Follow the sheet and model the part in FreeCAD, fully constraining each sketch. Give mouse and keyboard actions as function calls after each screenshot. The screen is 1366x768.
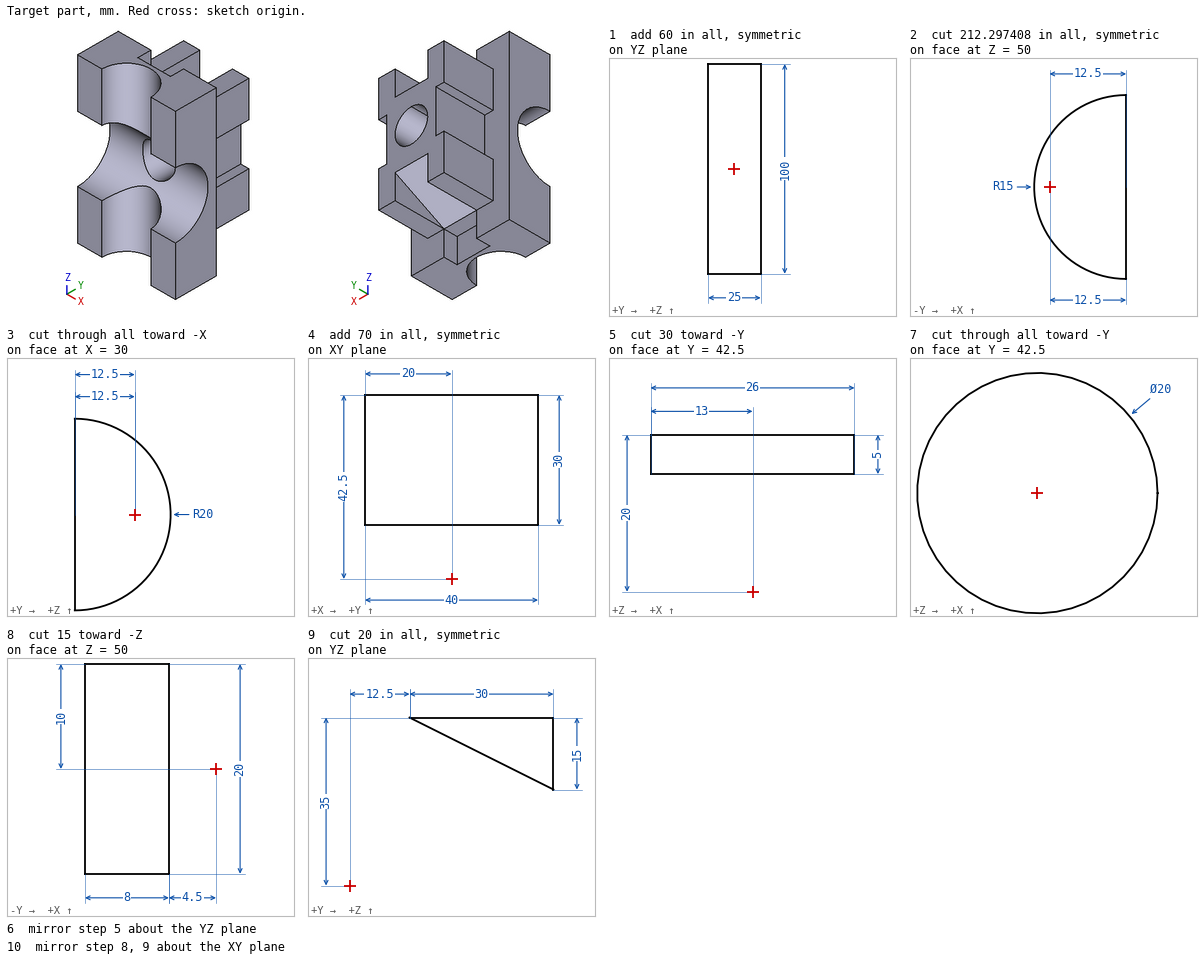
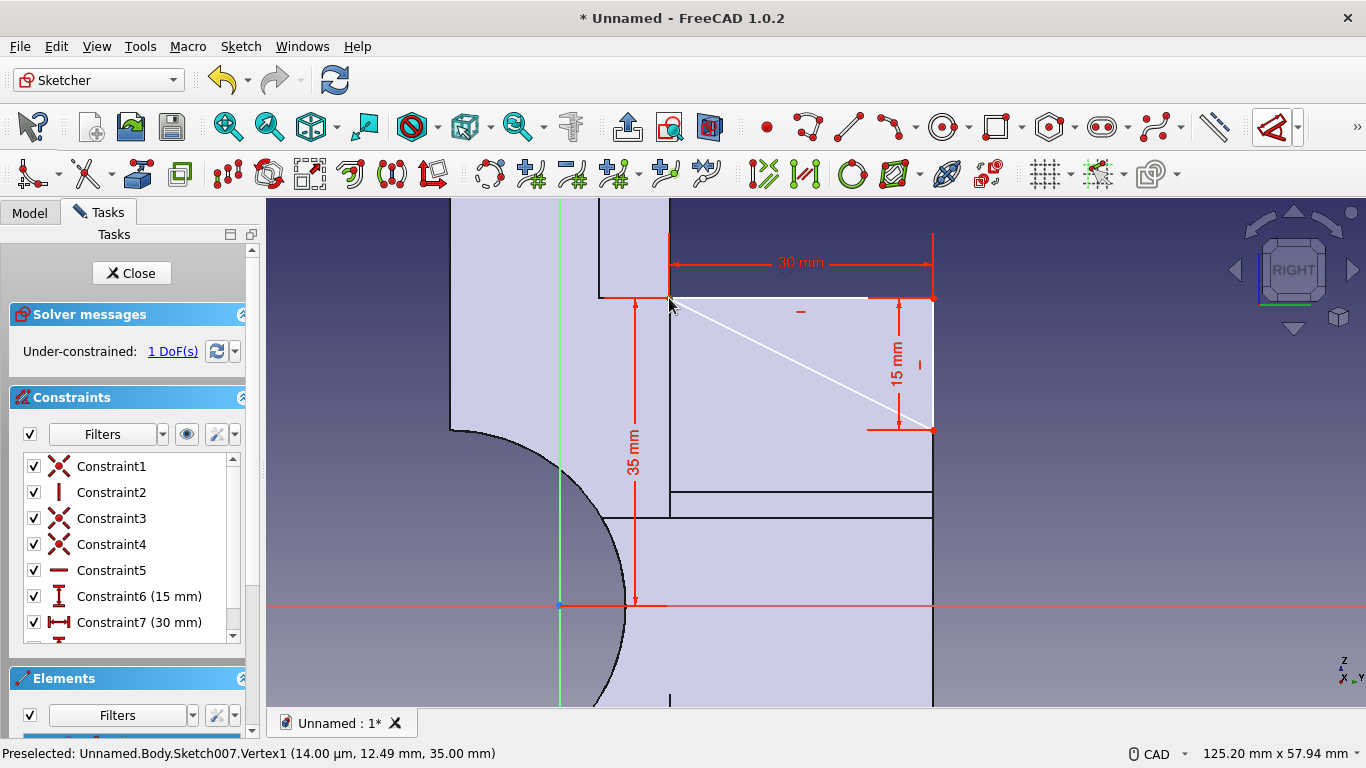
key(l)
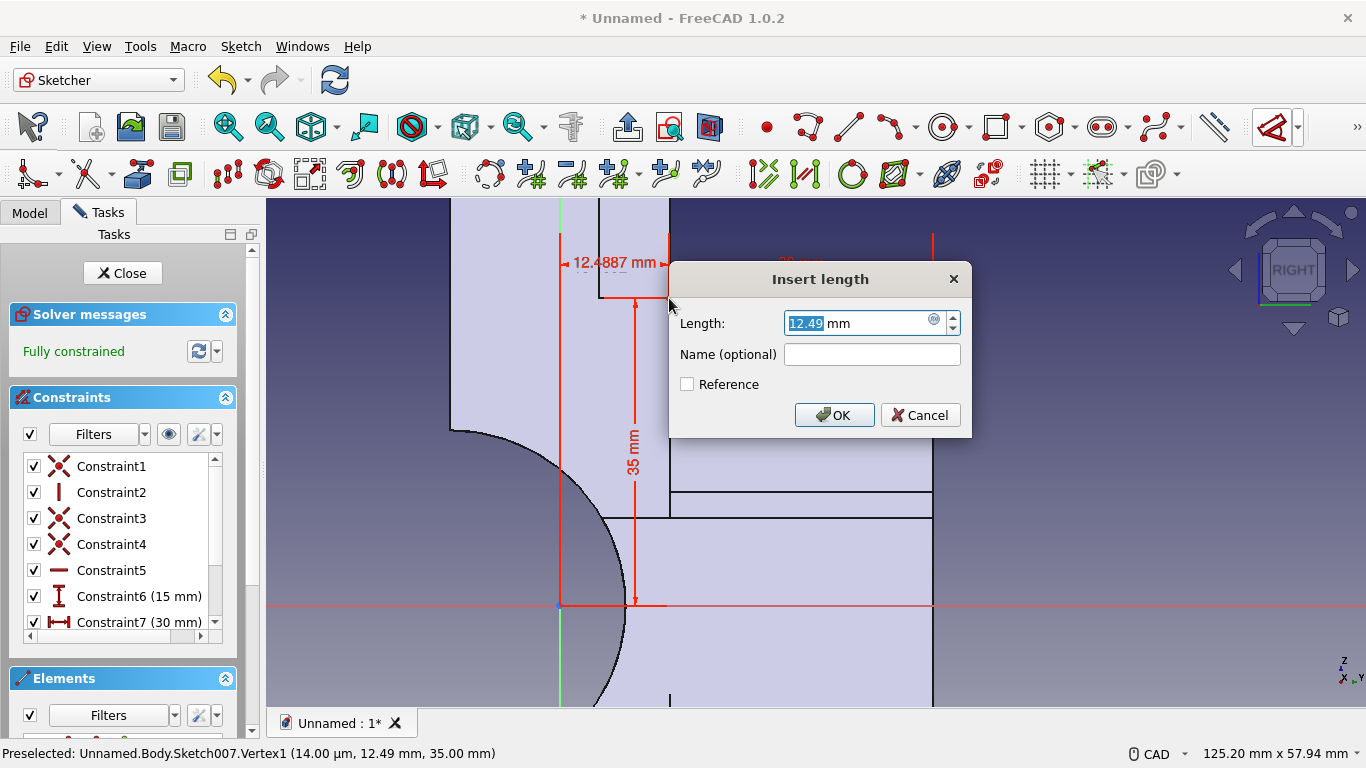
text(12.5)
key(Return)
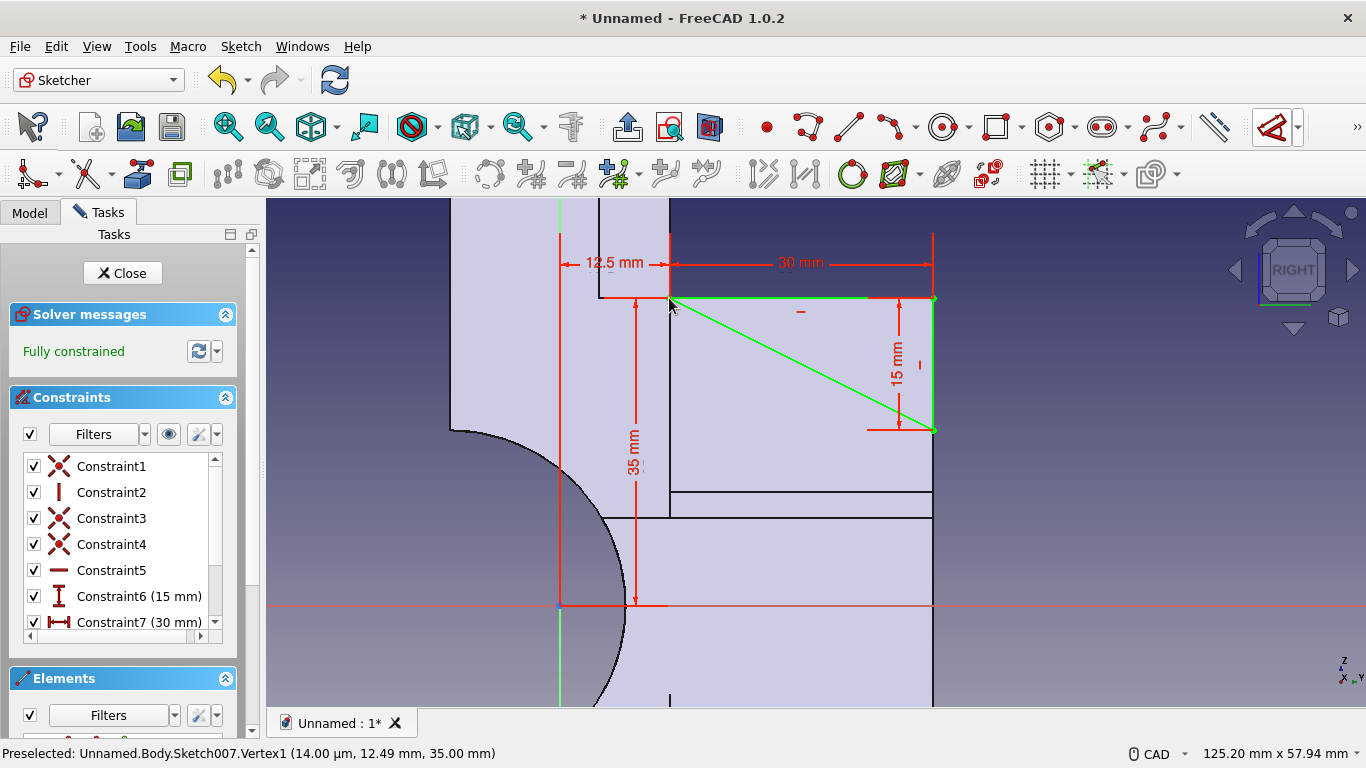
click(123, 273)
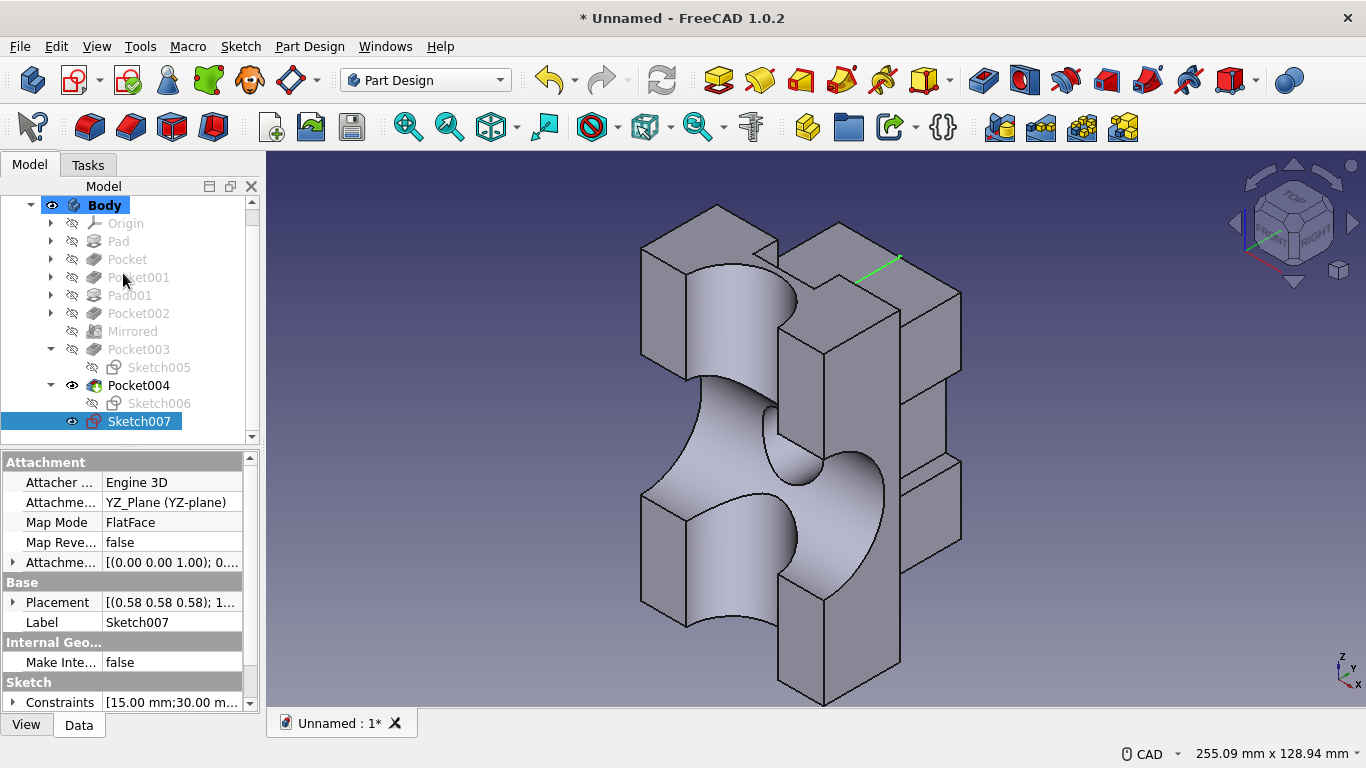
click(984, 80)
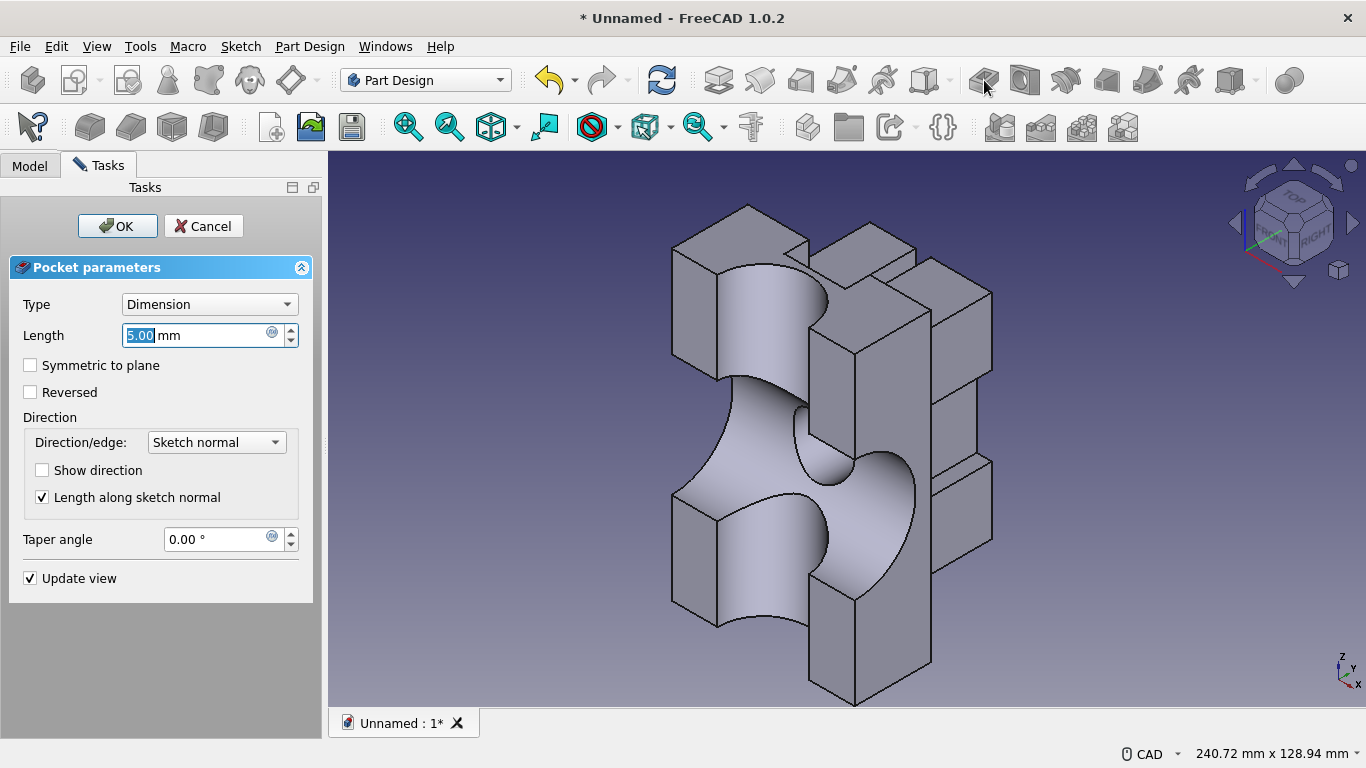
text(20)
key(Tab)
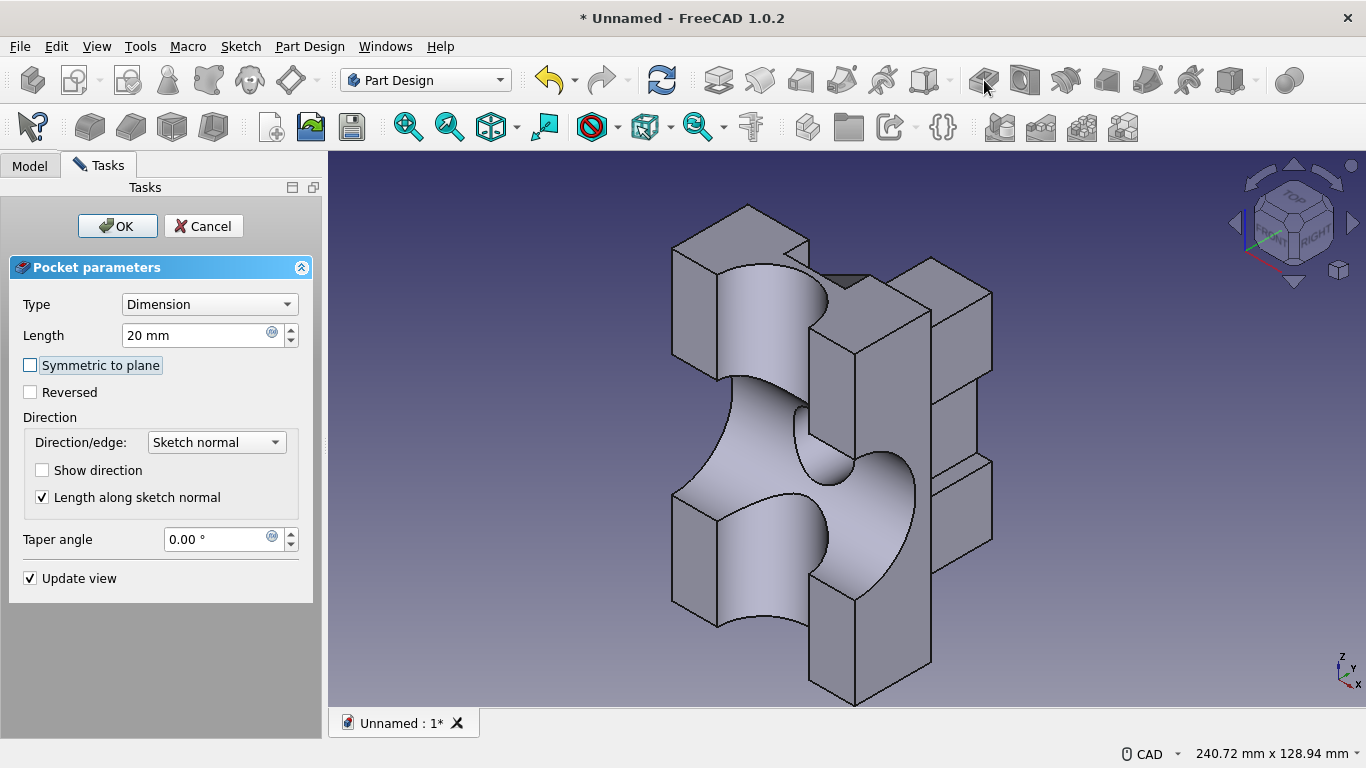
click(31, 365)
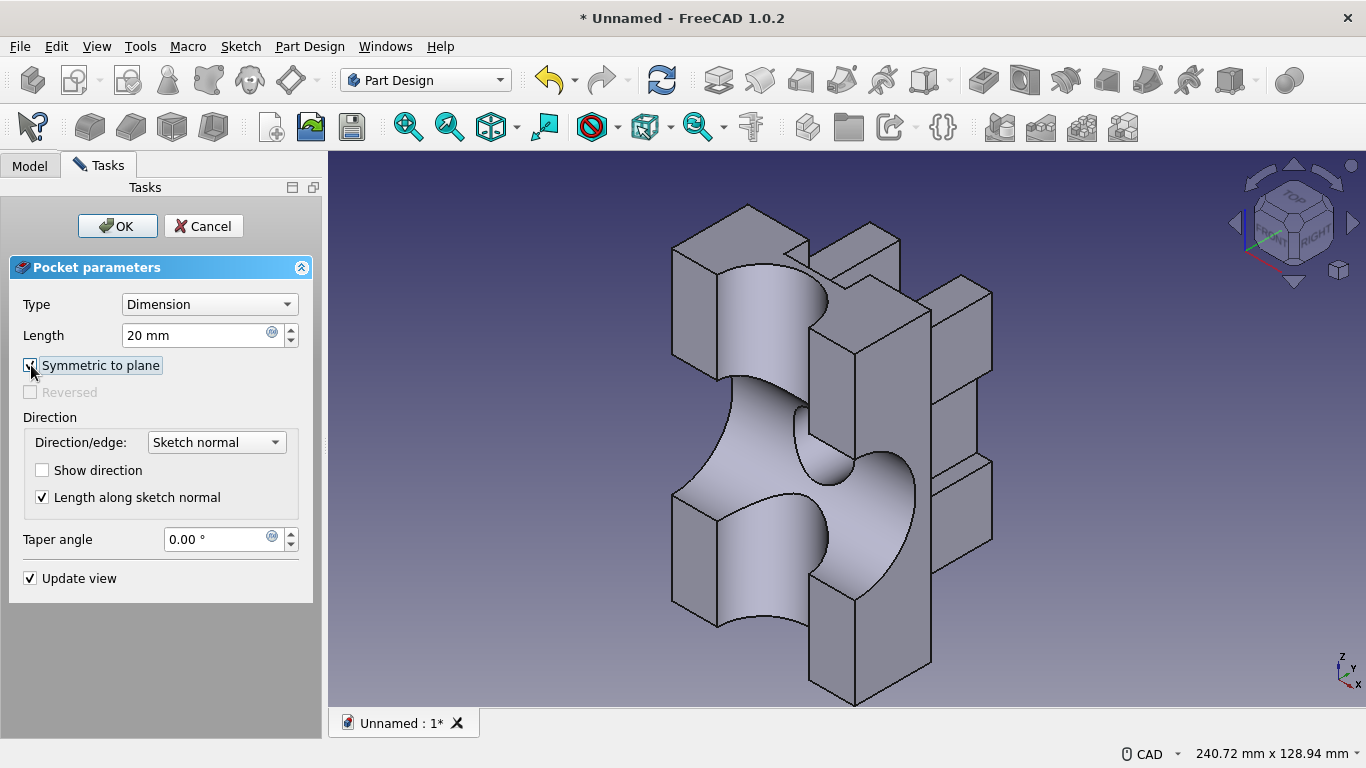
click(118, 226)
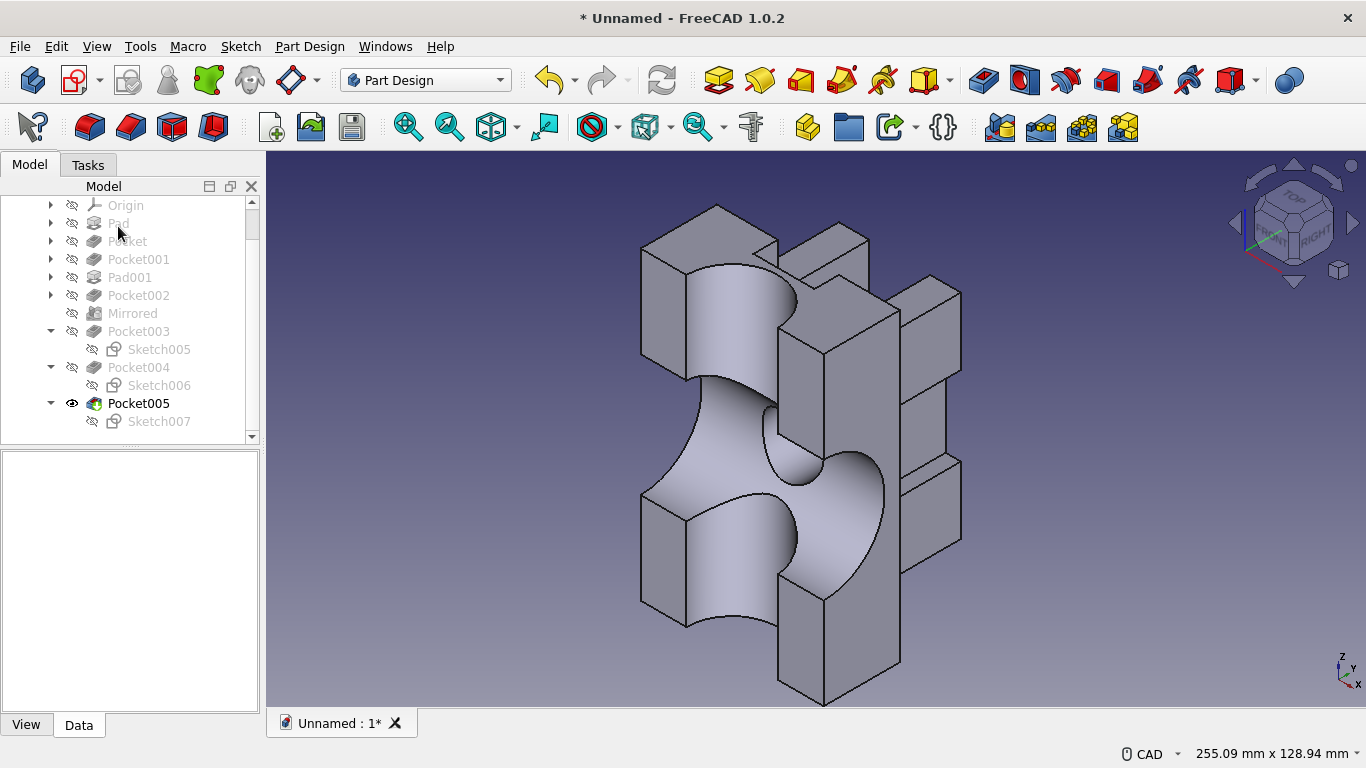
click(117, 367)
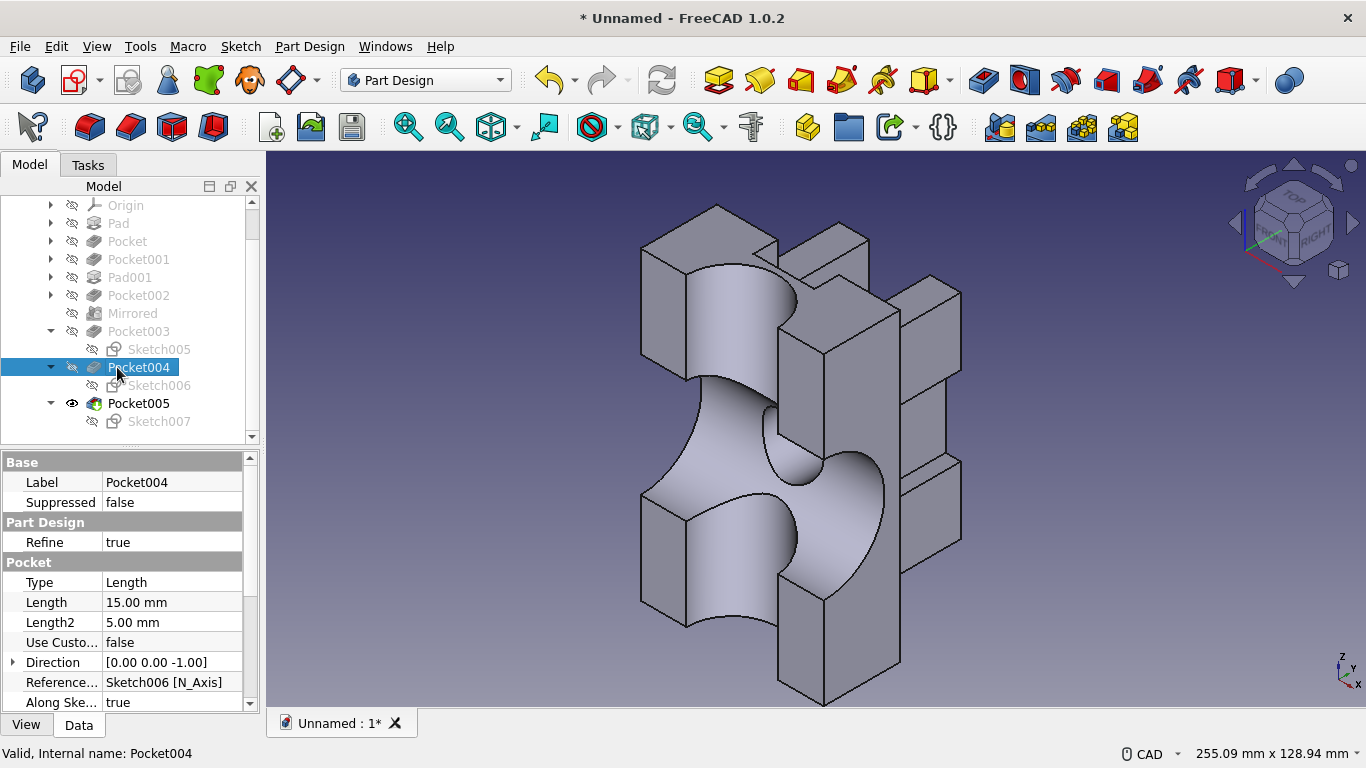
click(117, 403, ctrl)